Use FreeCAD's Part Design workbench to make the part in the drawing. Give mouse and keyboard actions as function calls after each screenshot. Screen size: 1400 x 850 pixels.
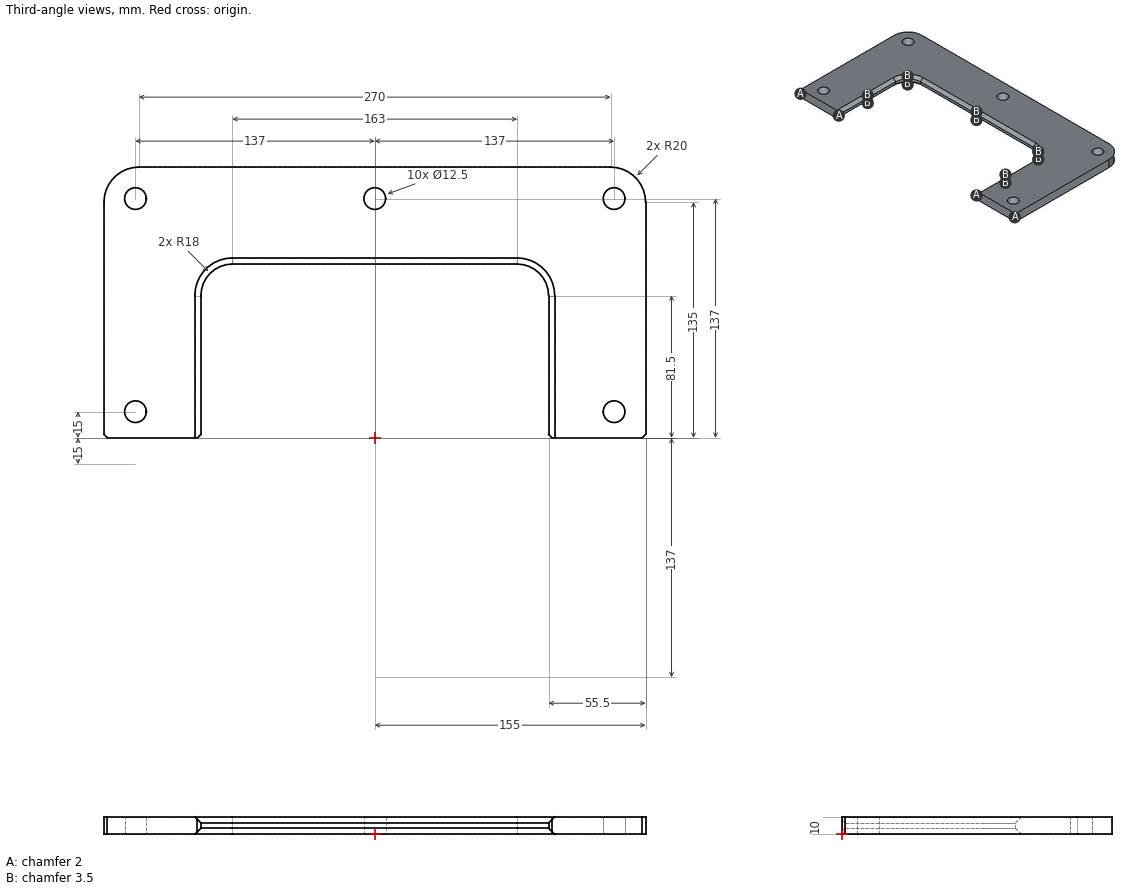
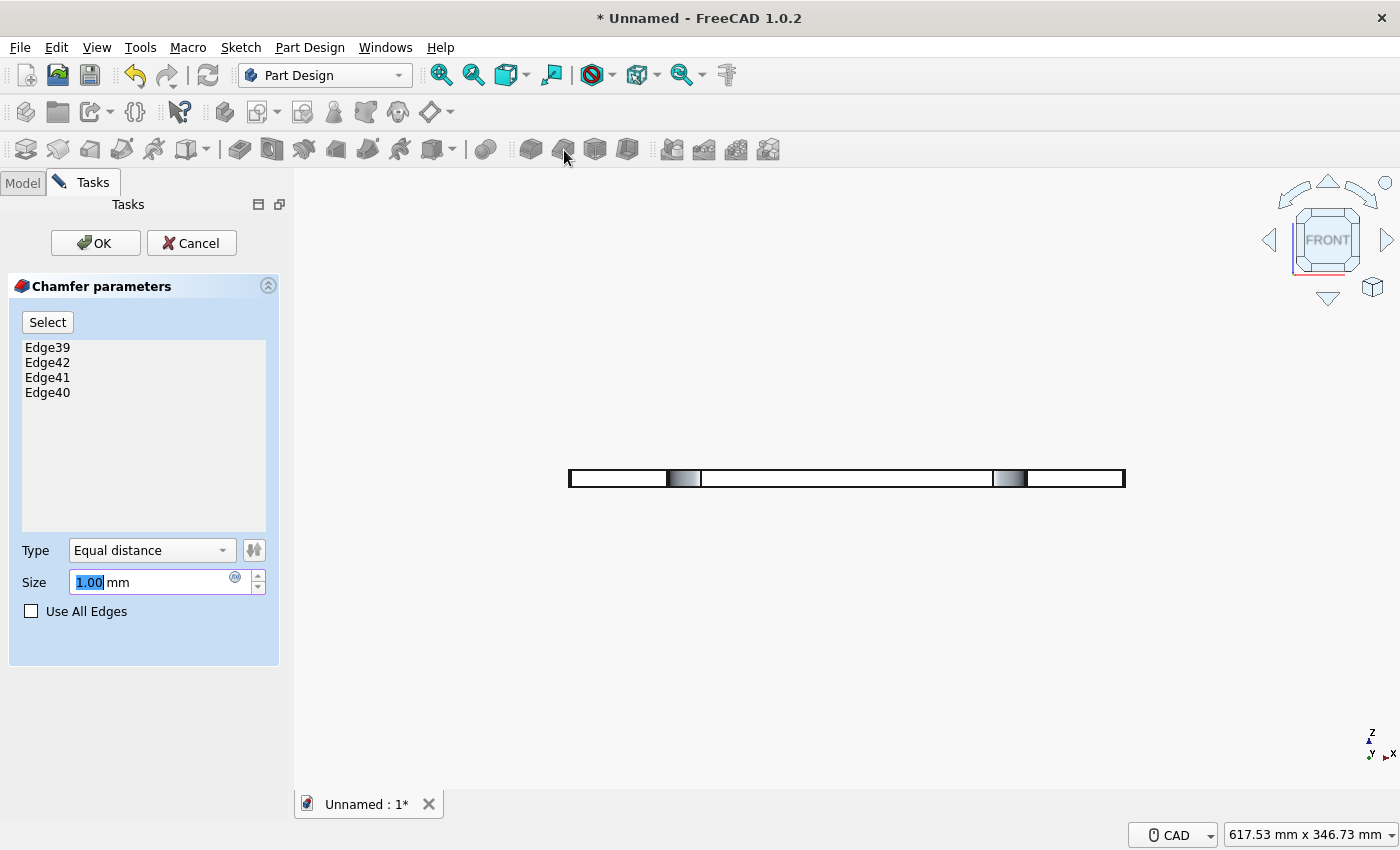
text(2)
key(Tab)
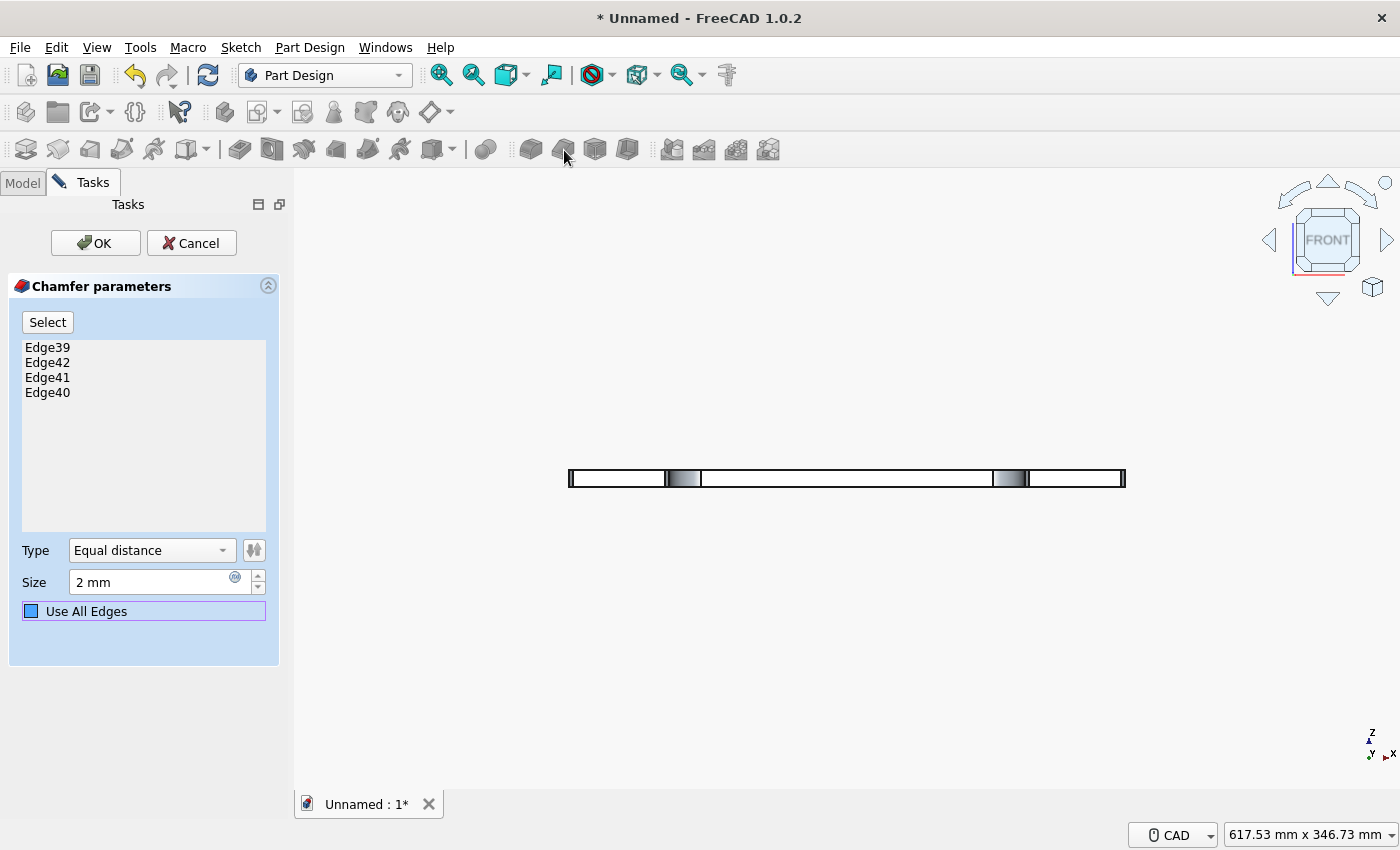
click(96, 243)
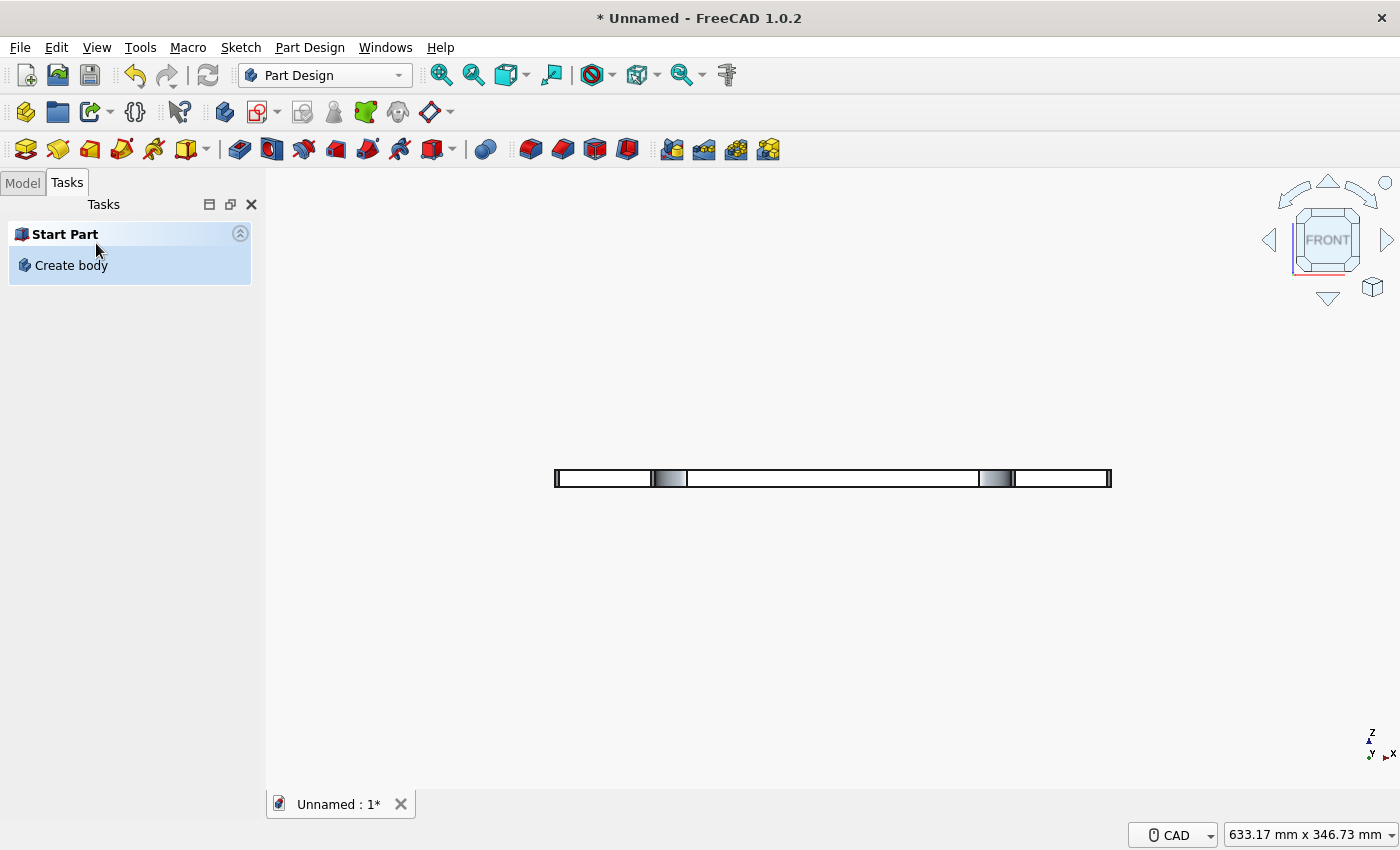
click(1002, 486)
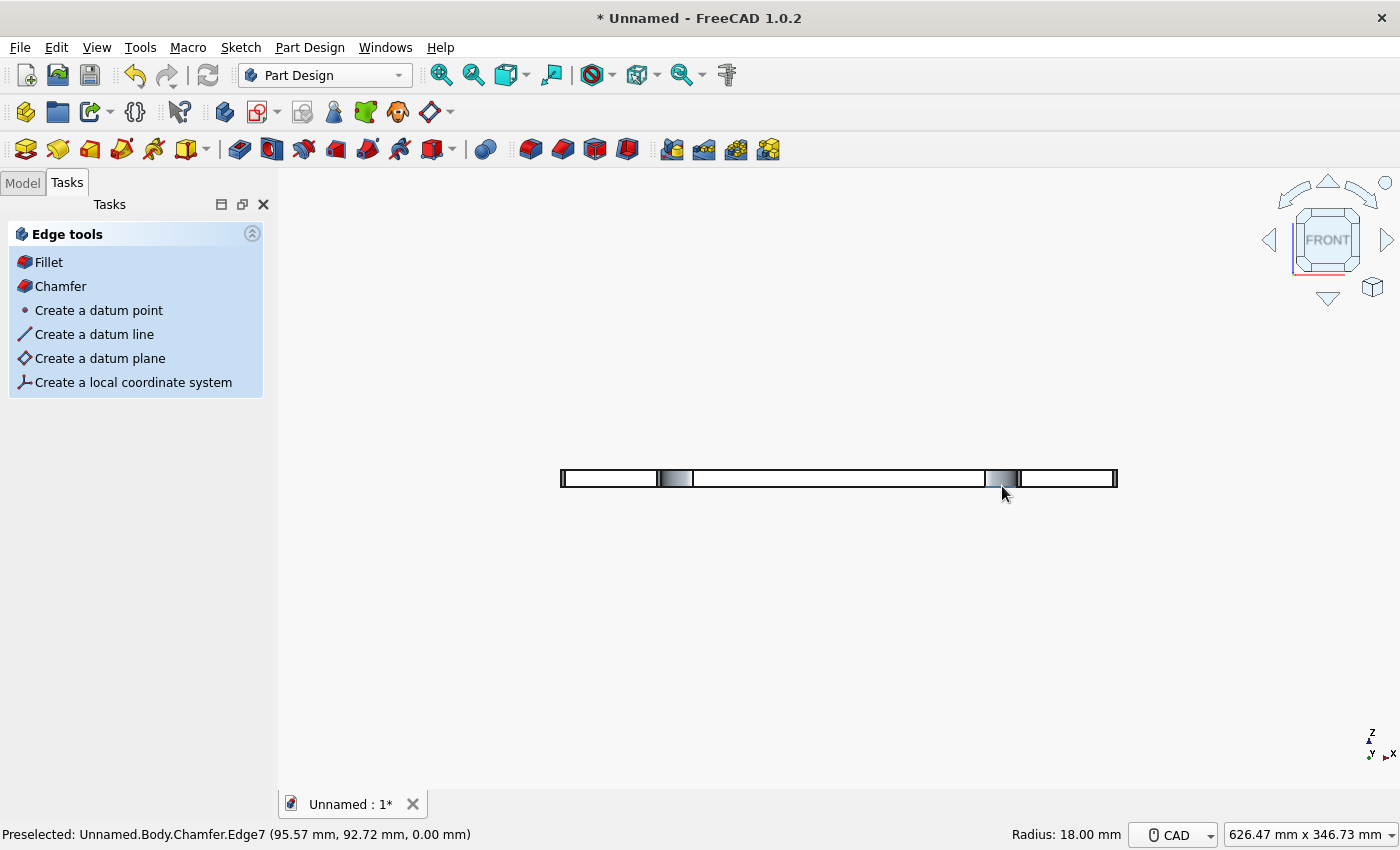
click(839, 486, ctrl)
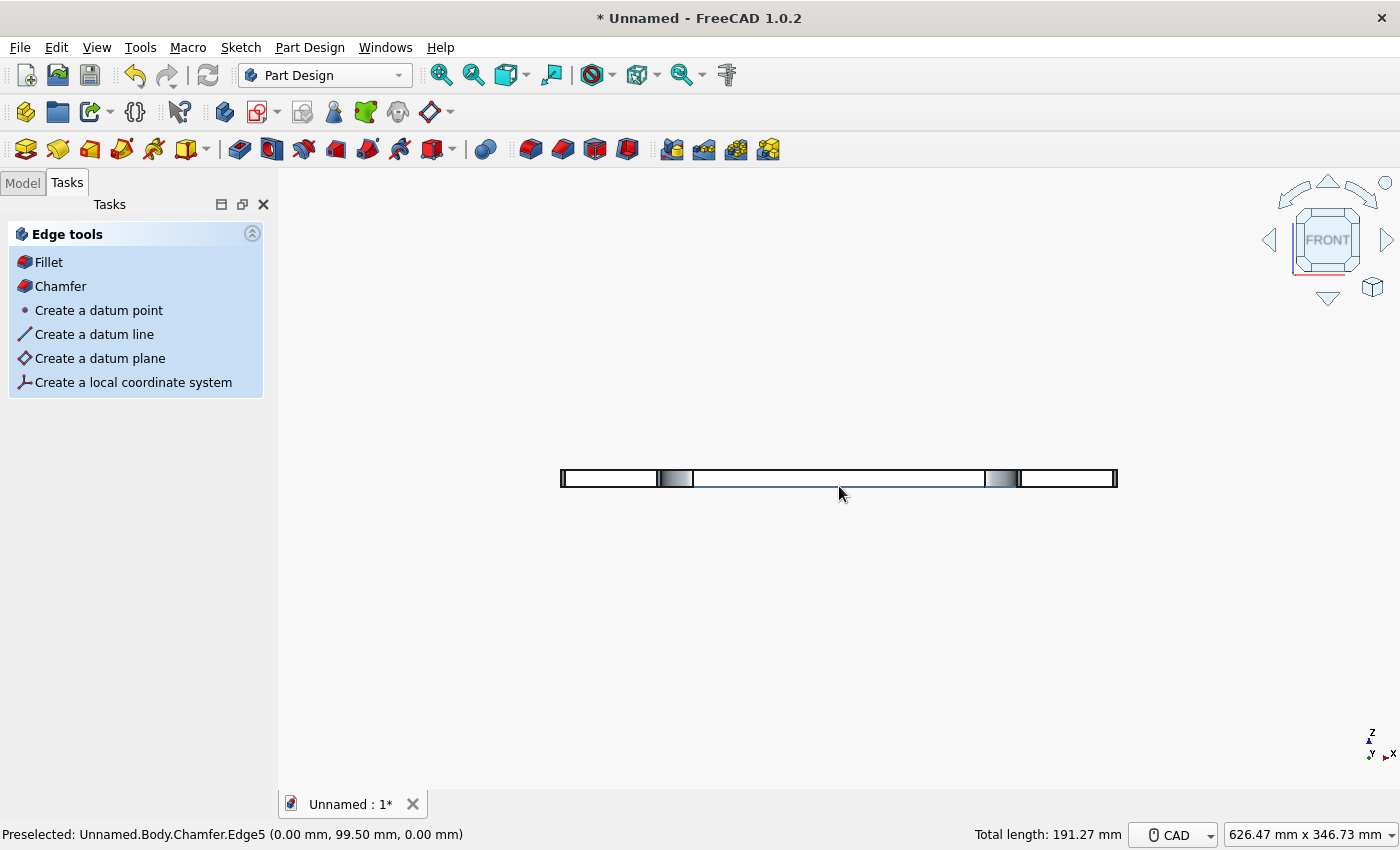
click(670, 486, ctrl)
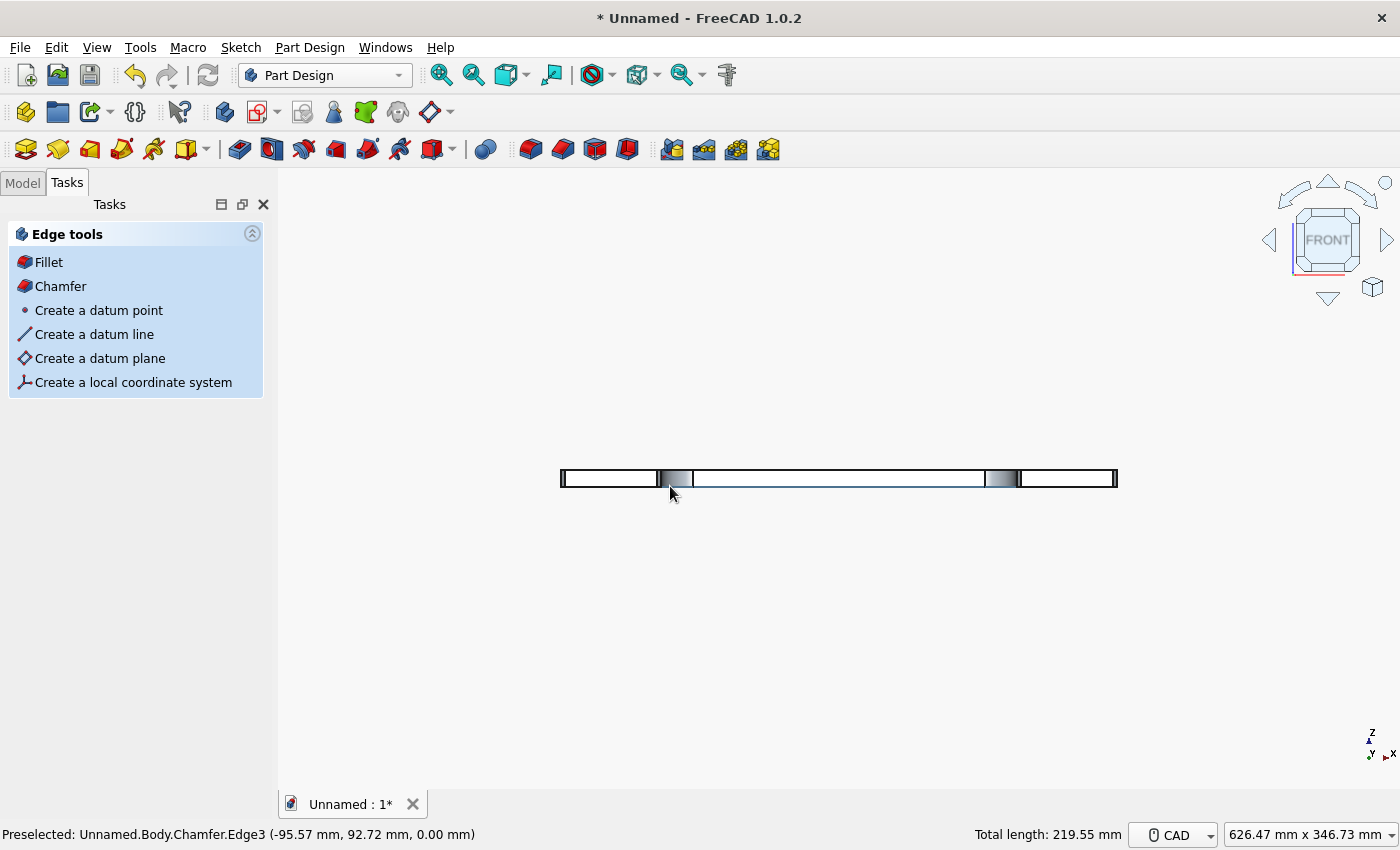
click(1008, 469, ctrl)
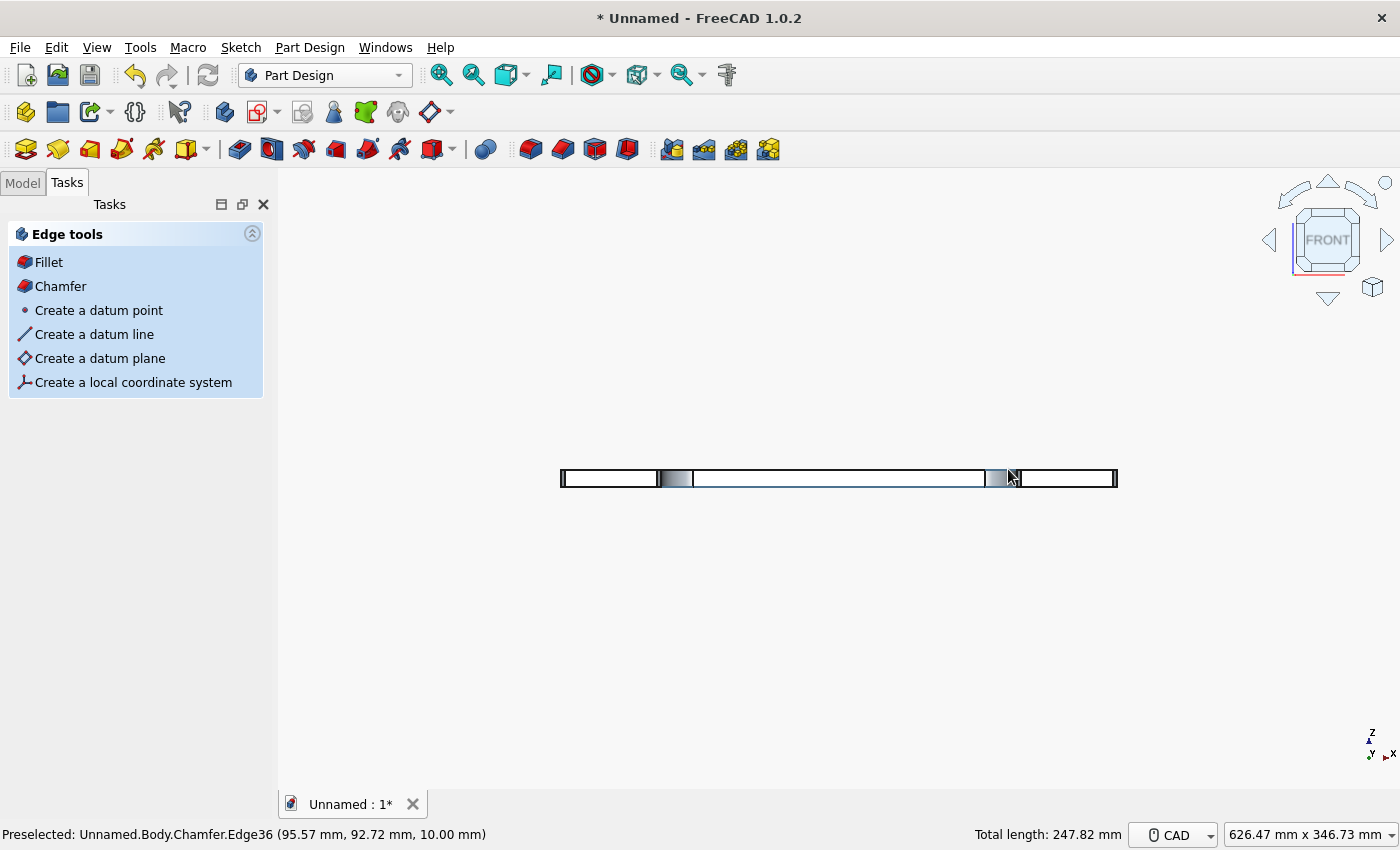
click(670, 469, ctrl)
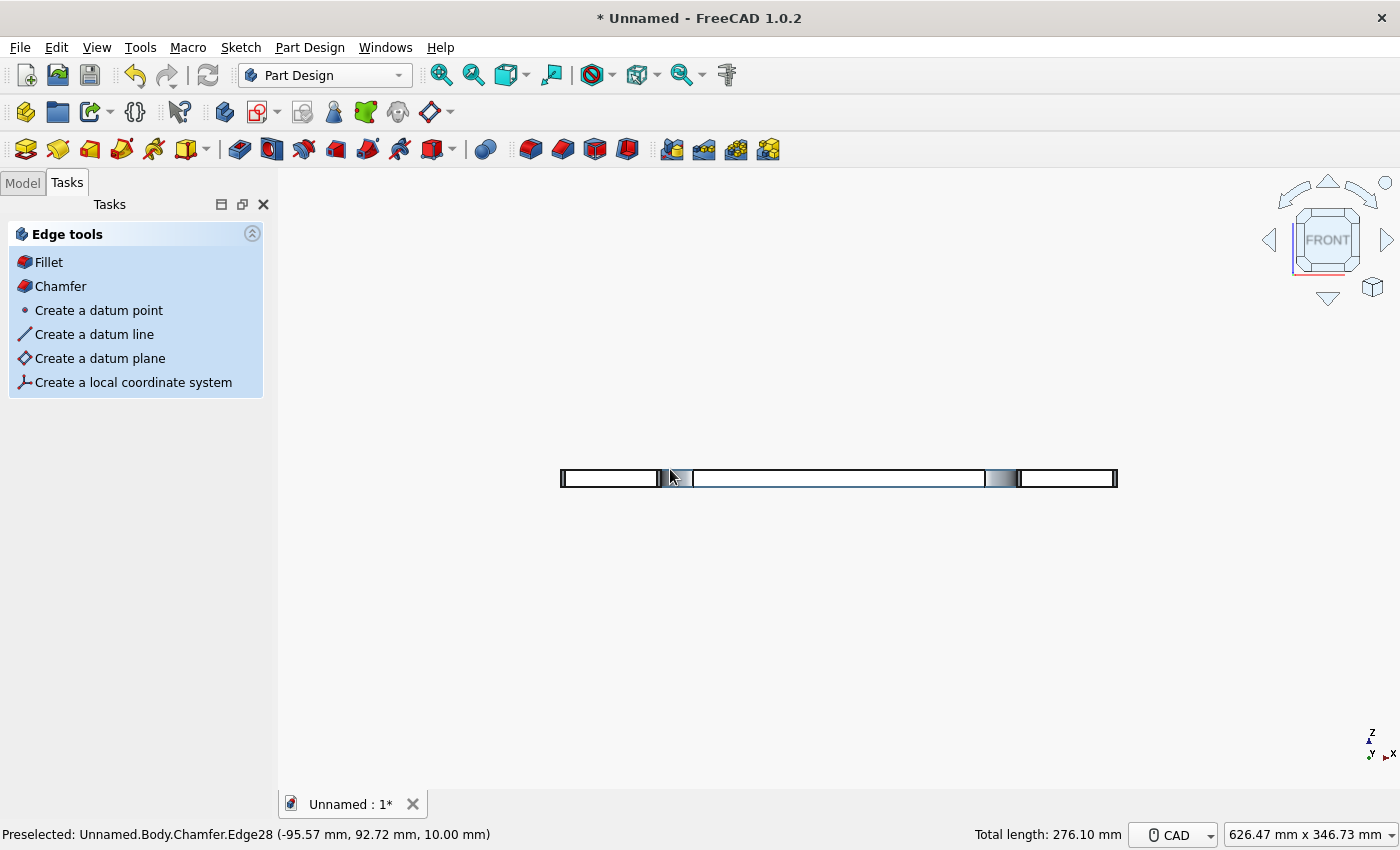
click(839, 469, ctrl)